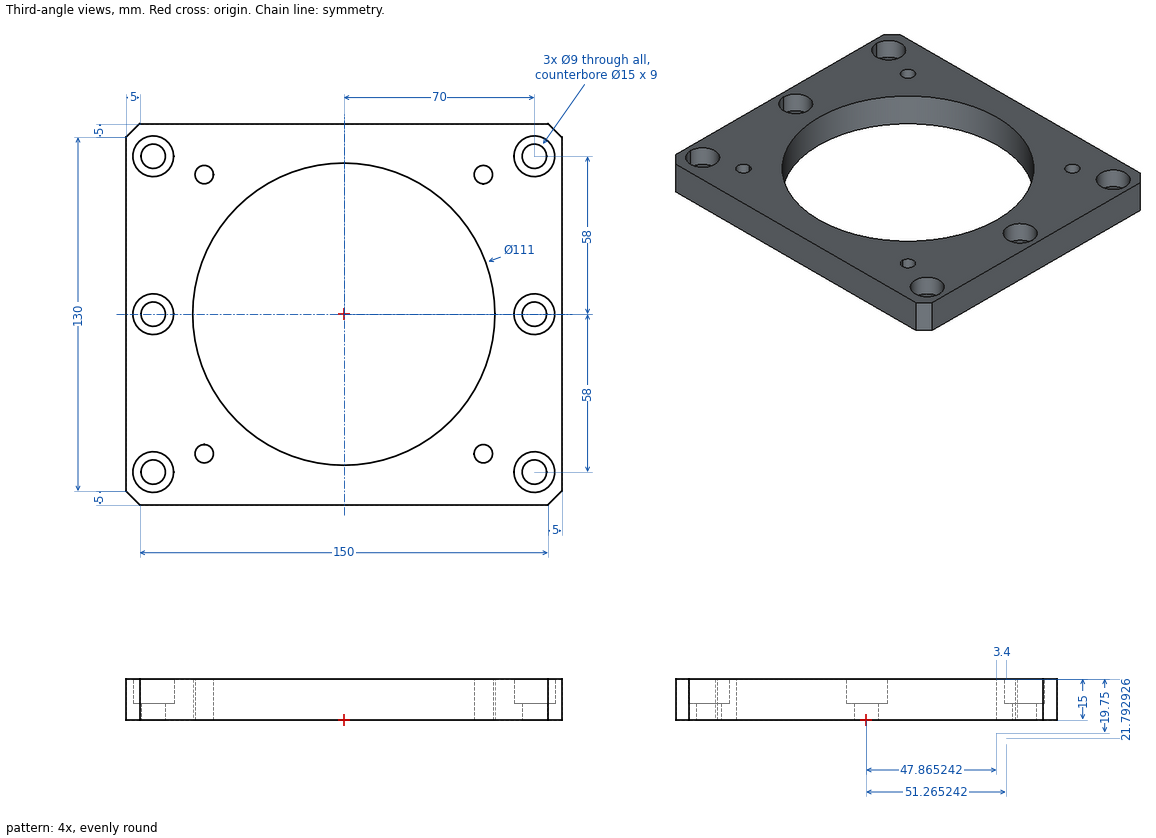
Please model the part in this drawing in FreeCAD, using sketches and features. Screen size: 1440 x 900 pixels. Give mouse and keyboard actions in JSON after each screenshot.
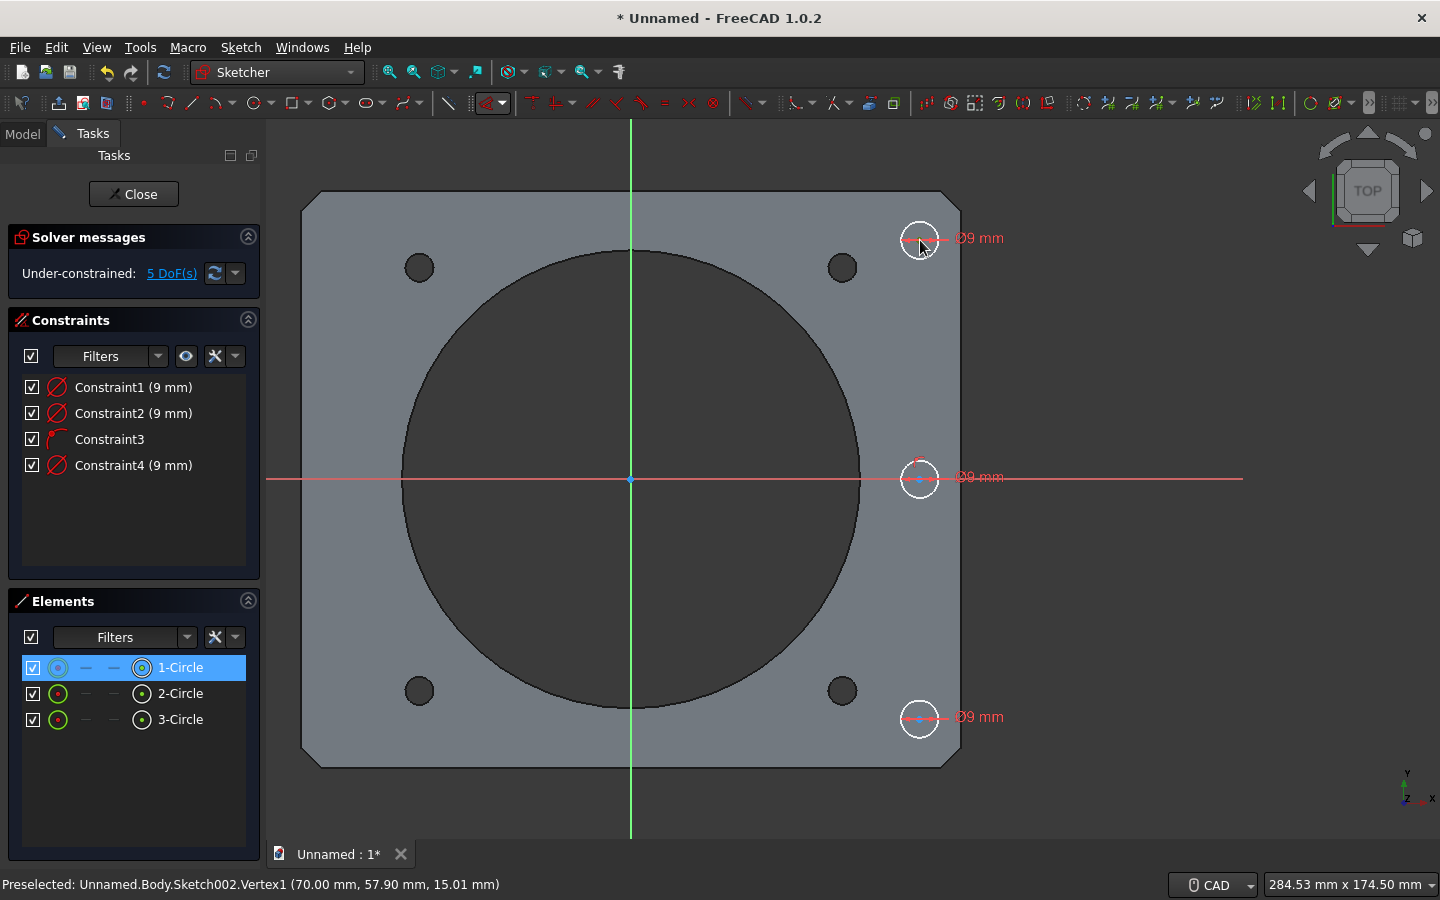
{"action": "left_click", "coordinate": [920, 479]}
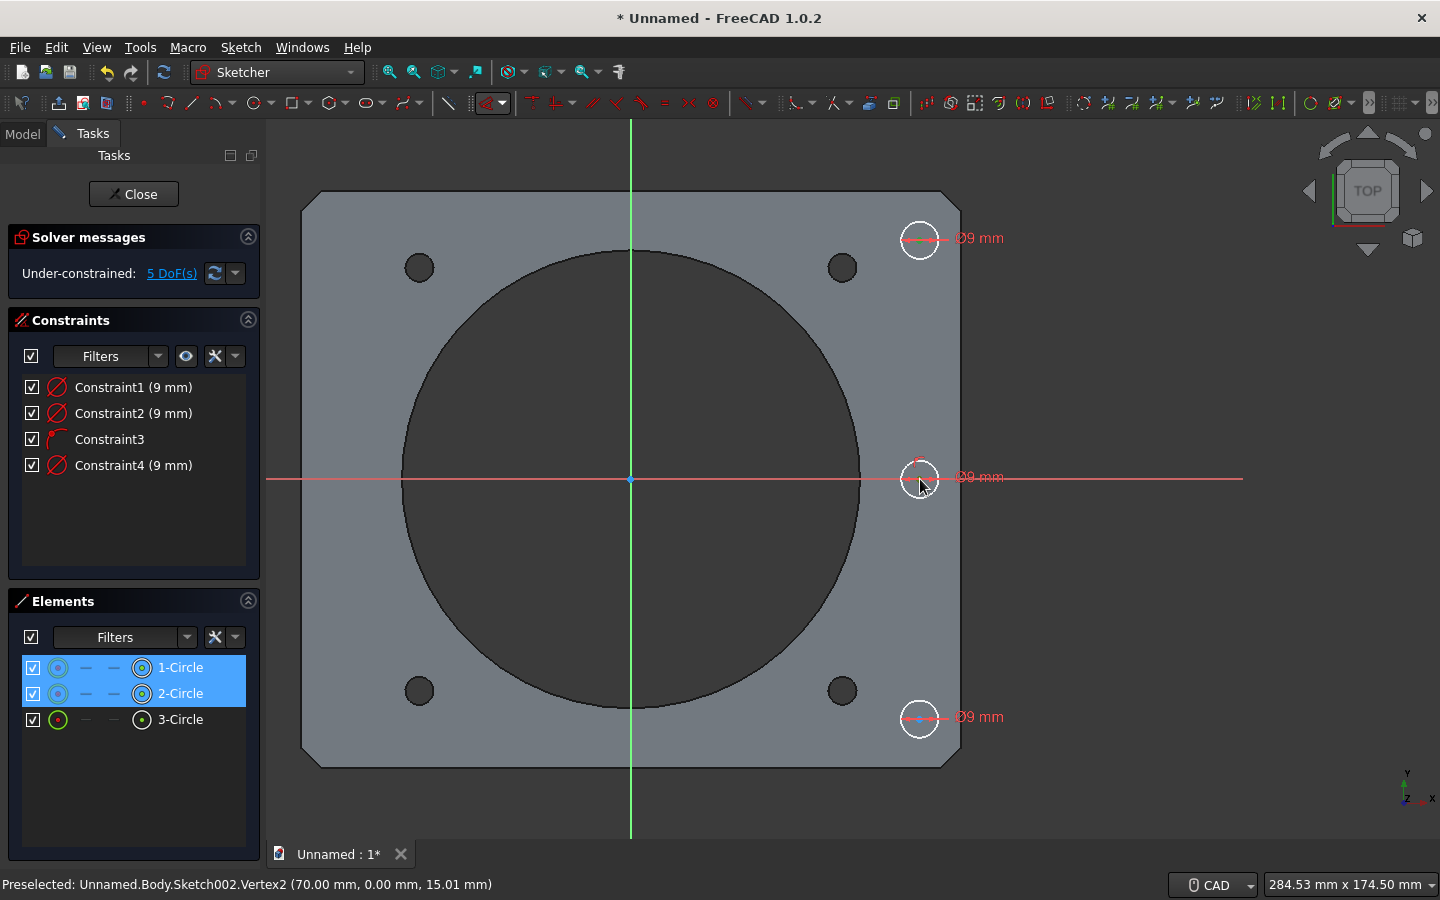
{"action": "key", "text": "v"}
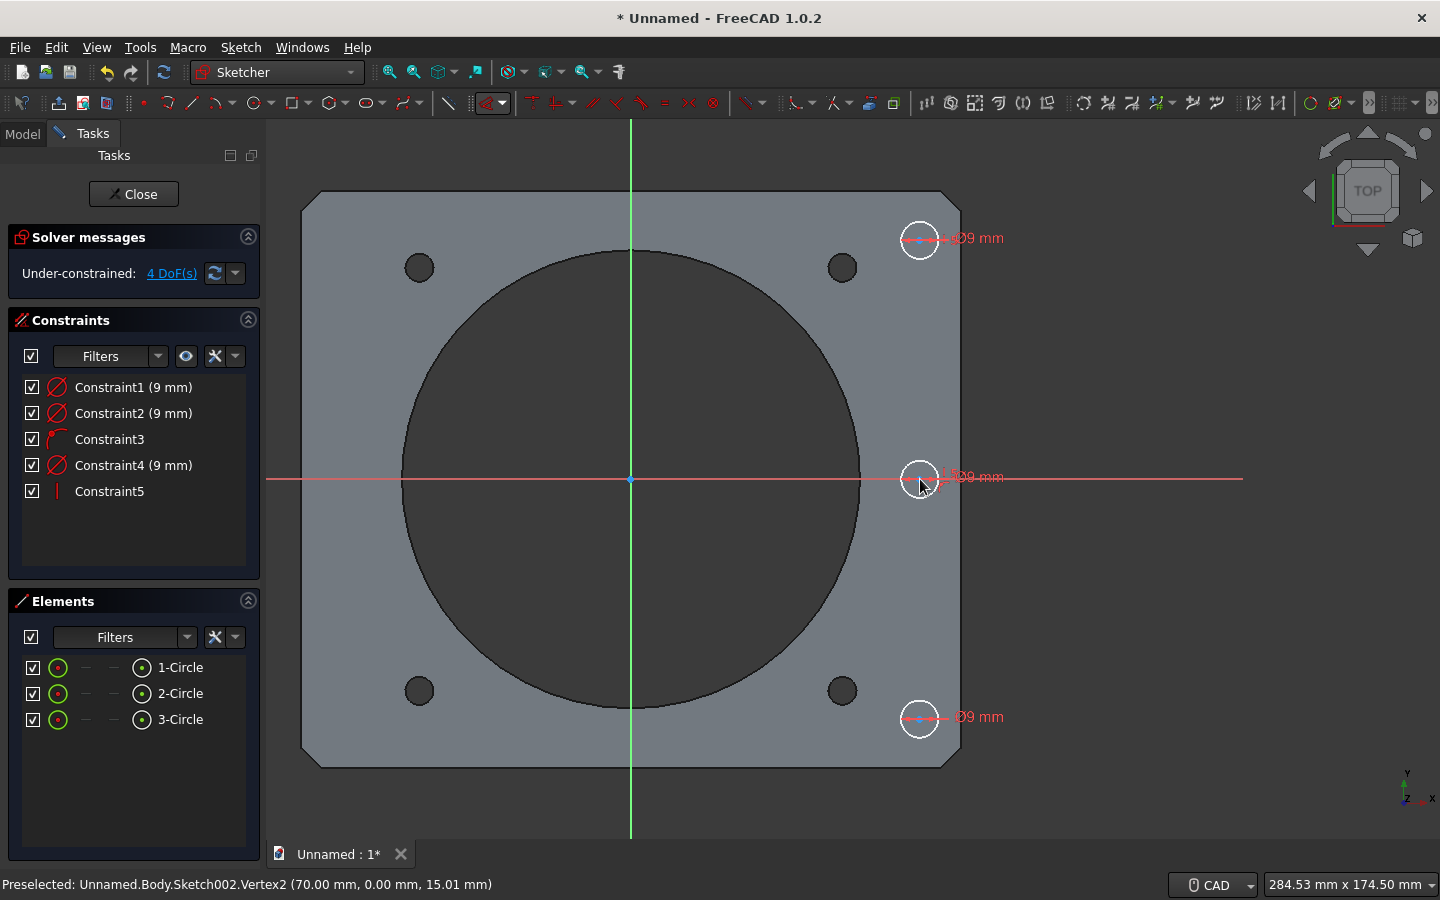
{"action": "left_click", "coordinate": [920, 479]}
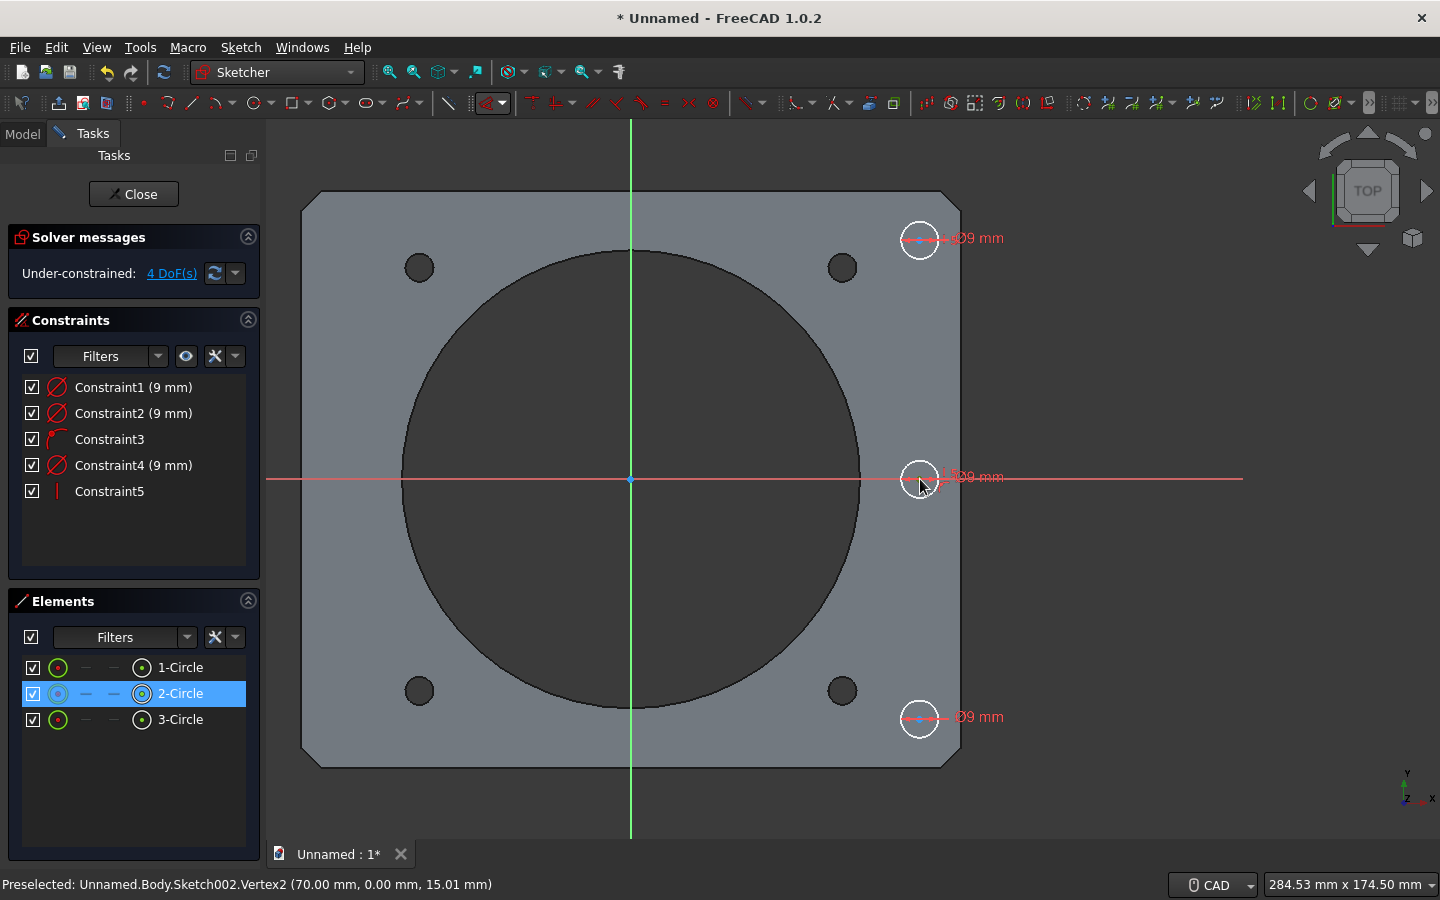
{"action": "left_click", "coordinate": [920, 719]}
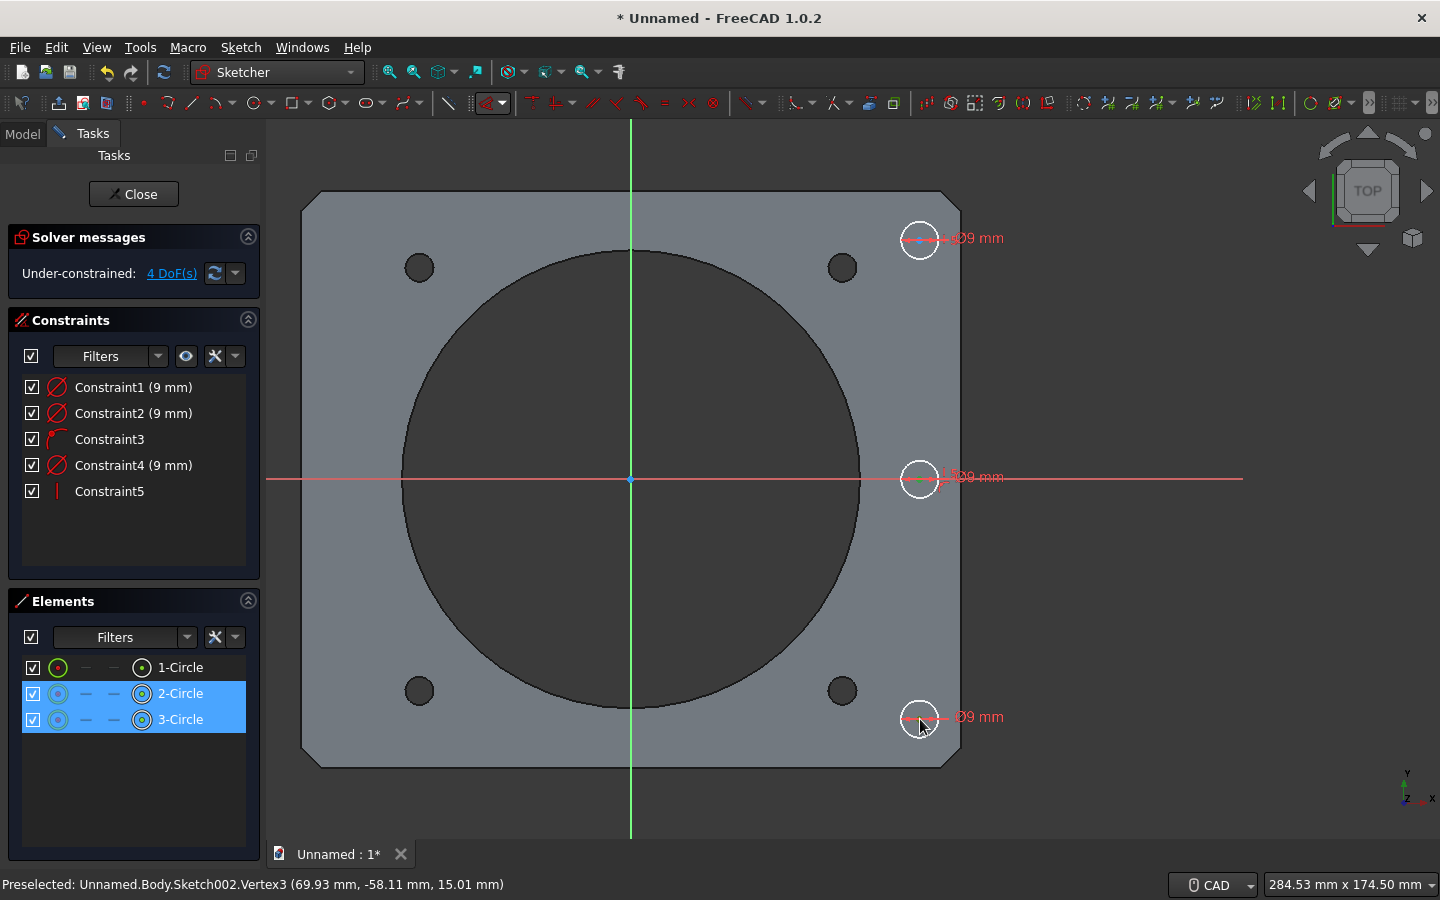
{"action": "key", "text": "v"}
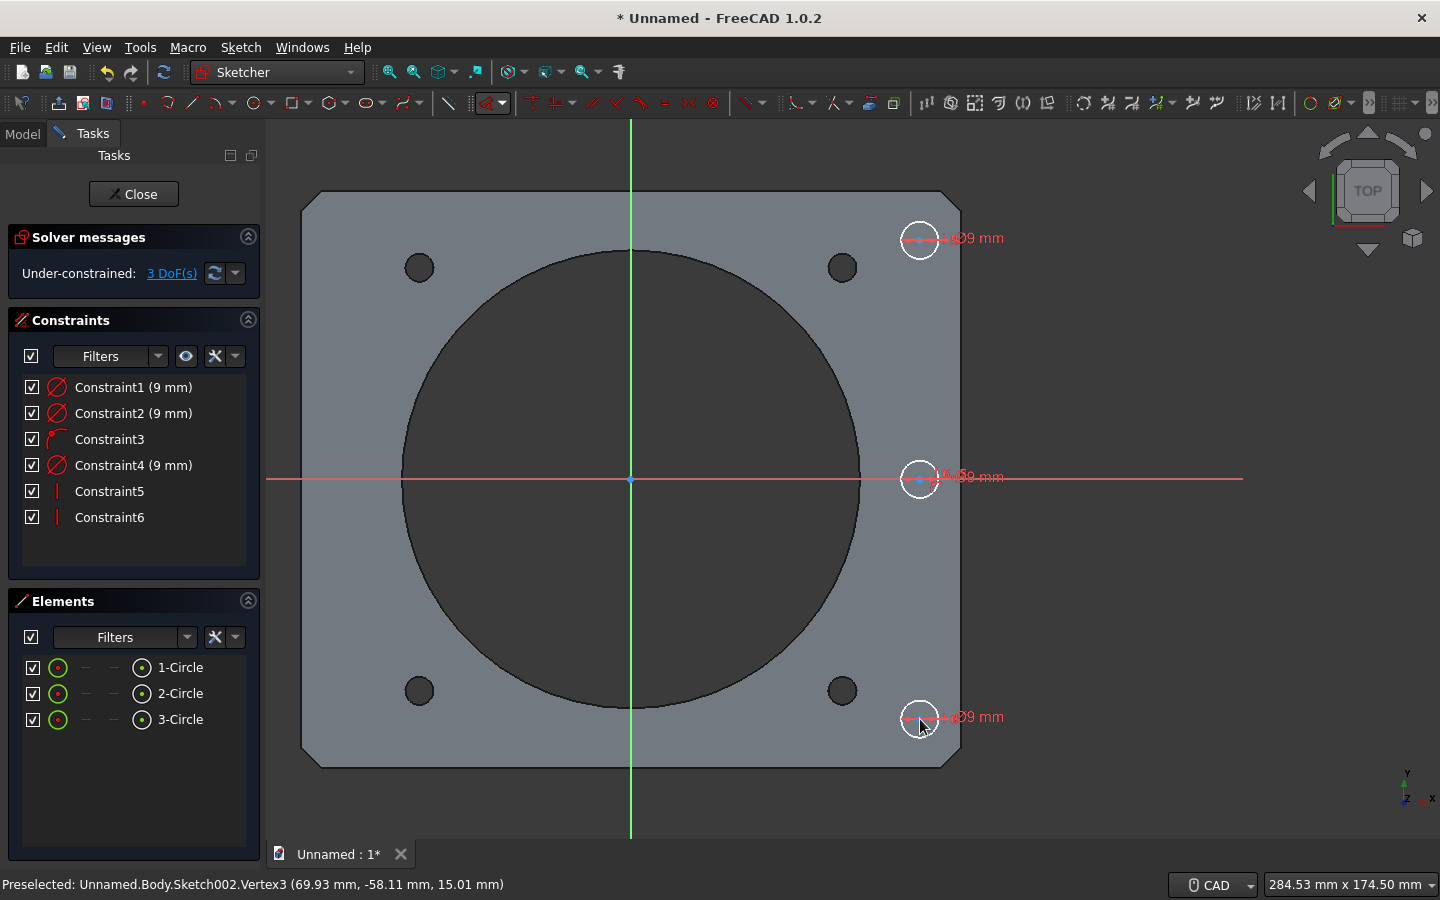
{"action": "left_click", "coordinate": [920, 240]}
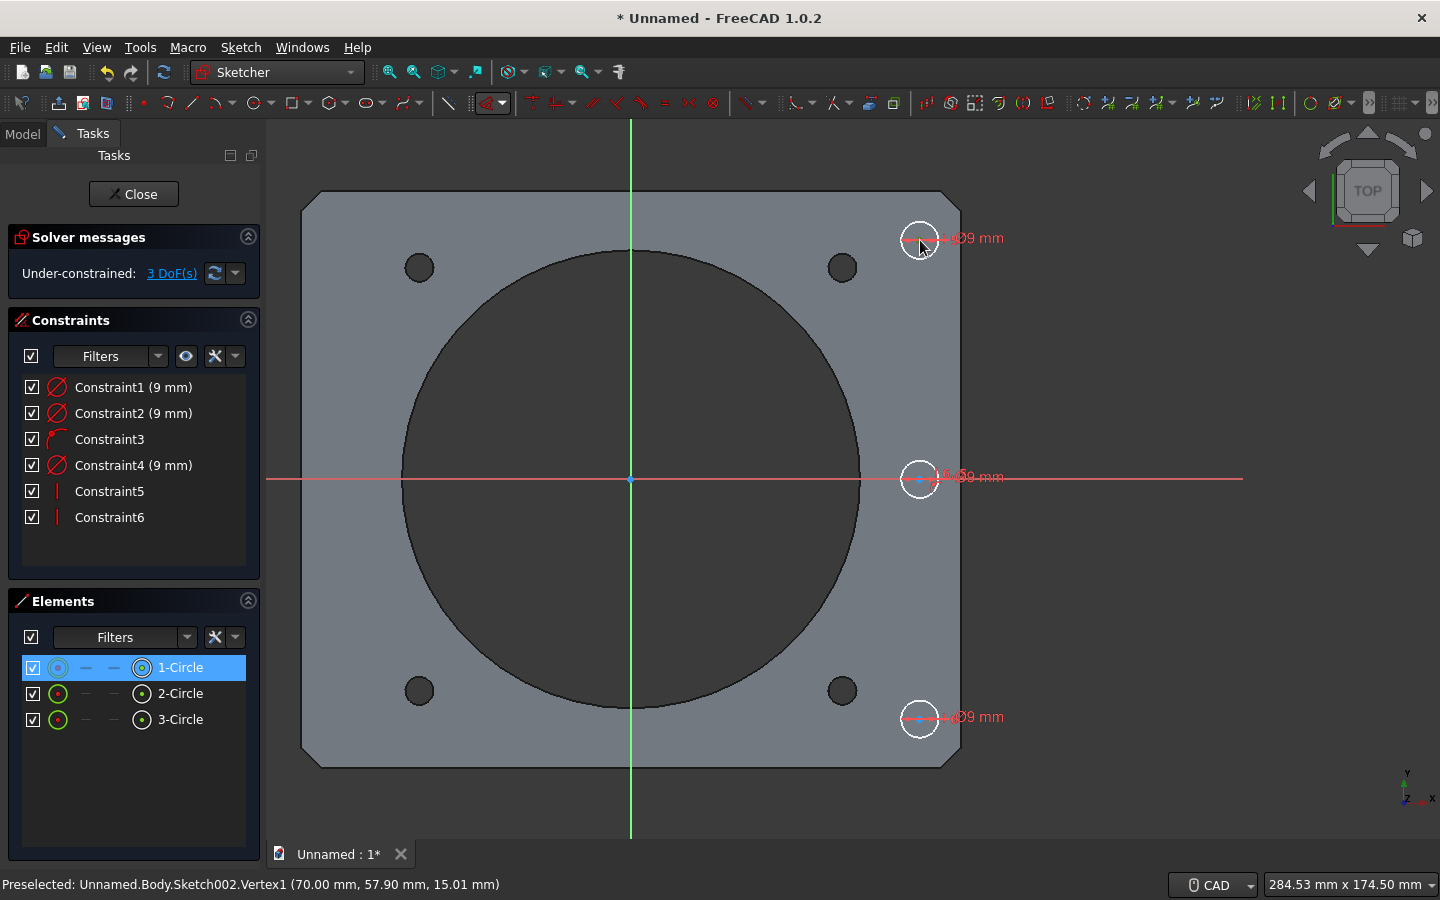
{"action": "key", "text": "l"}